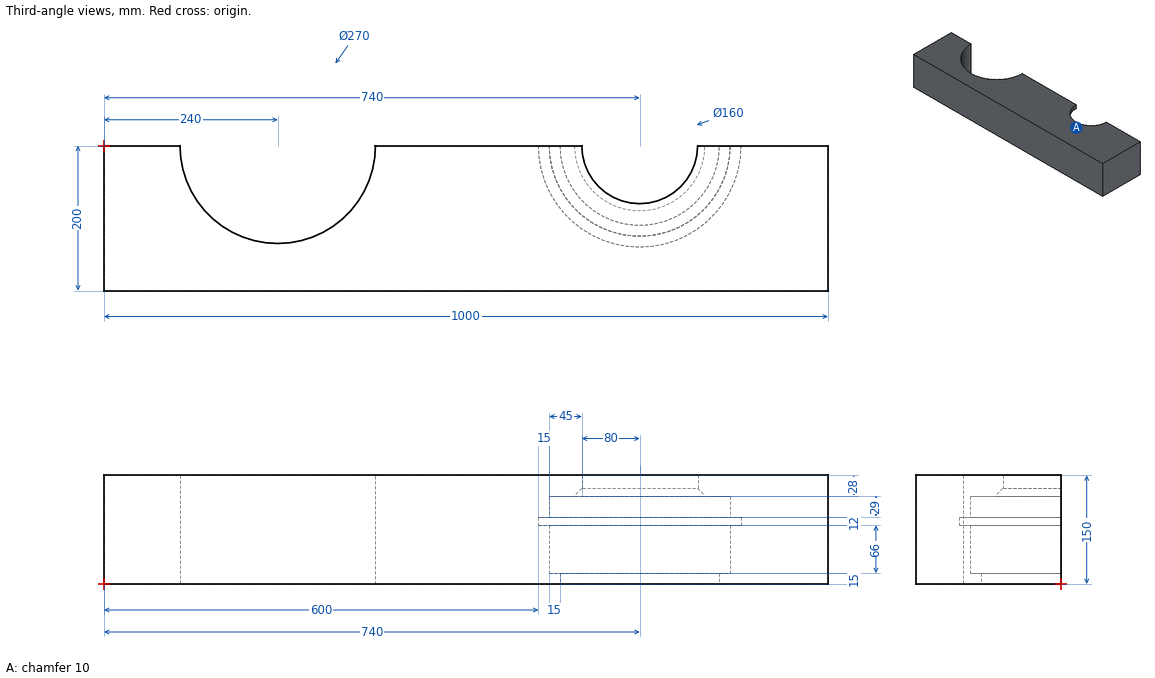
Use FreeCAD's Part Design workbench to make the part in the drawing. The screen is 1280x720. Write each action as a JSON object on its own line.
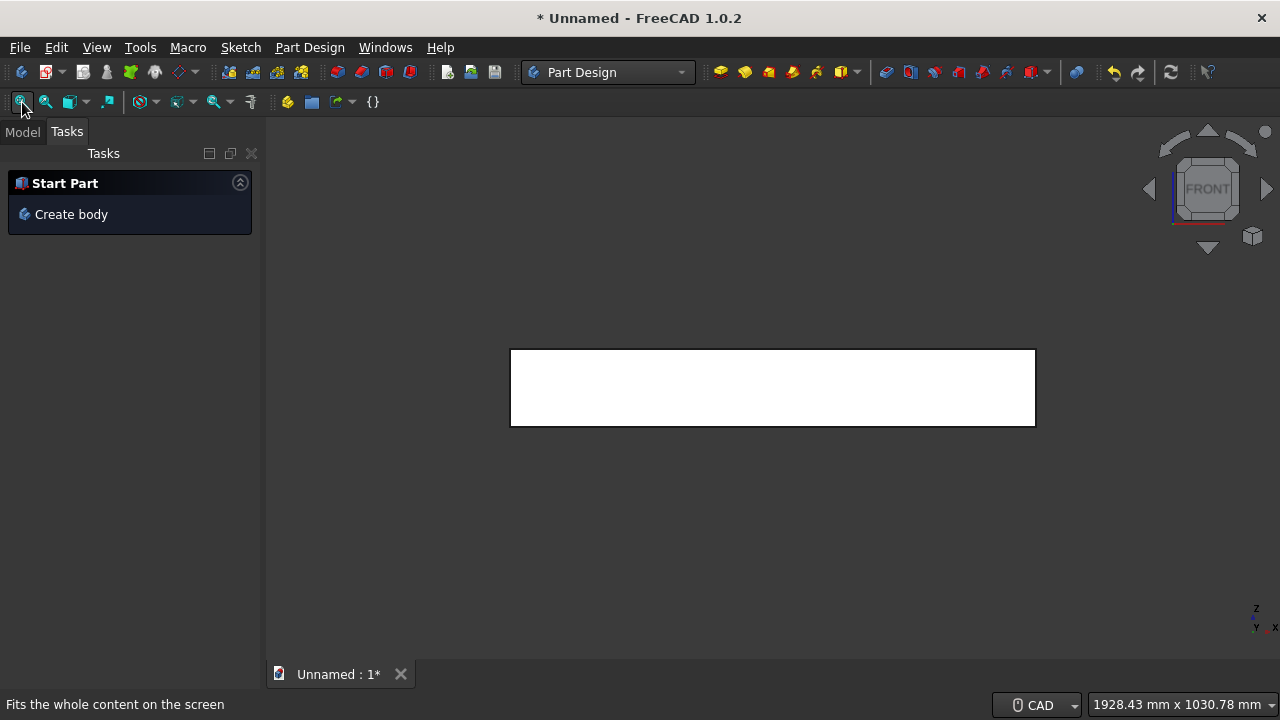
{"action": "key", "text": "3"}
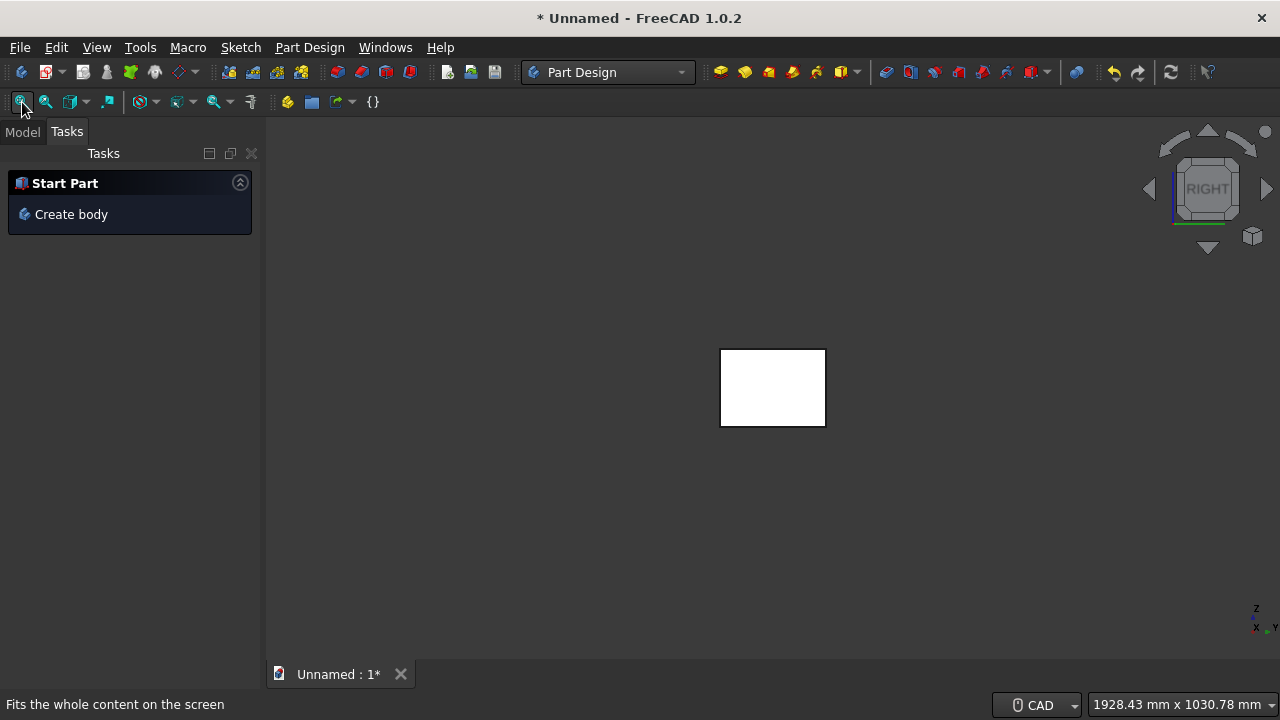
{"action": "left_click", "coordinate": [22, 102]}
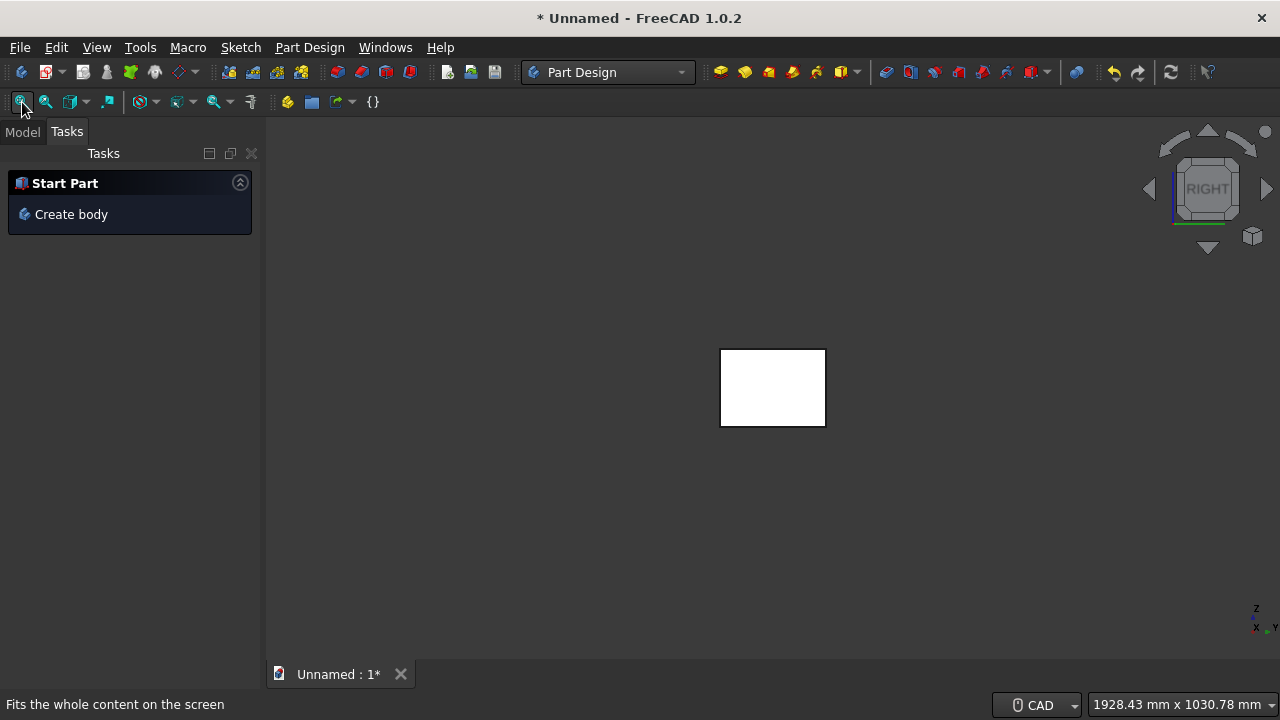
{"action": "key", "text": "5"}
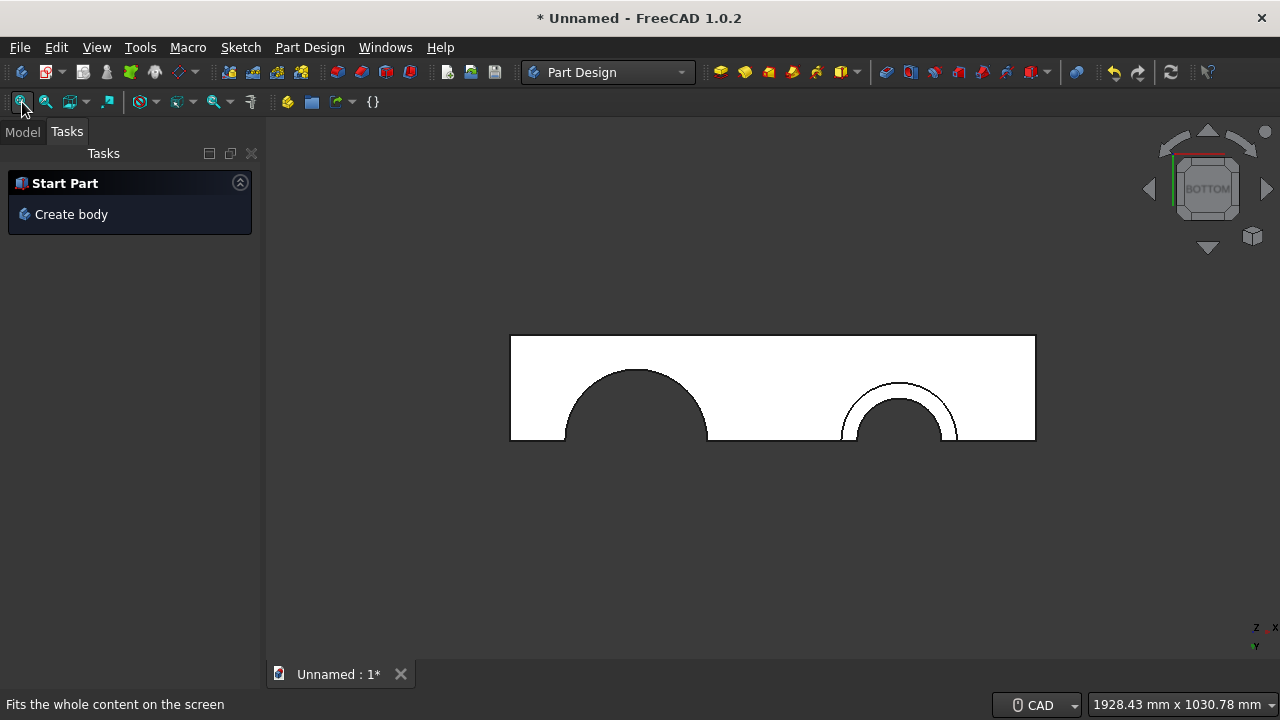
{"action": "left_click", "coordinate": [899, 398]}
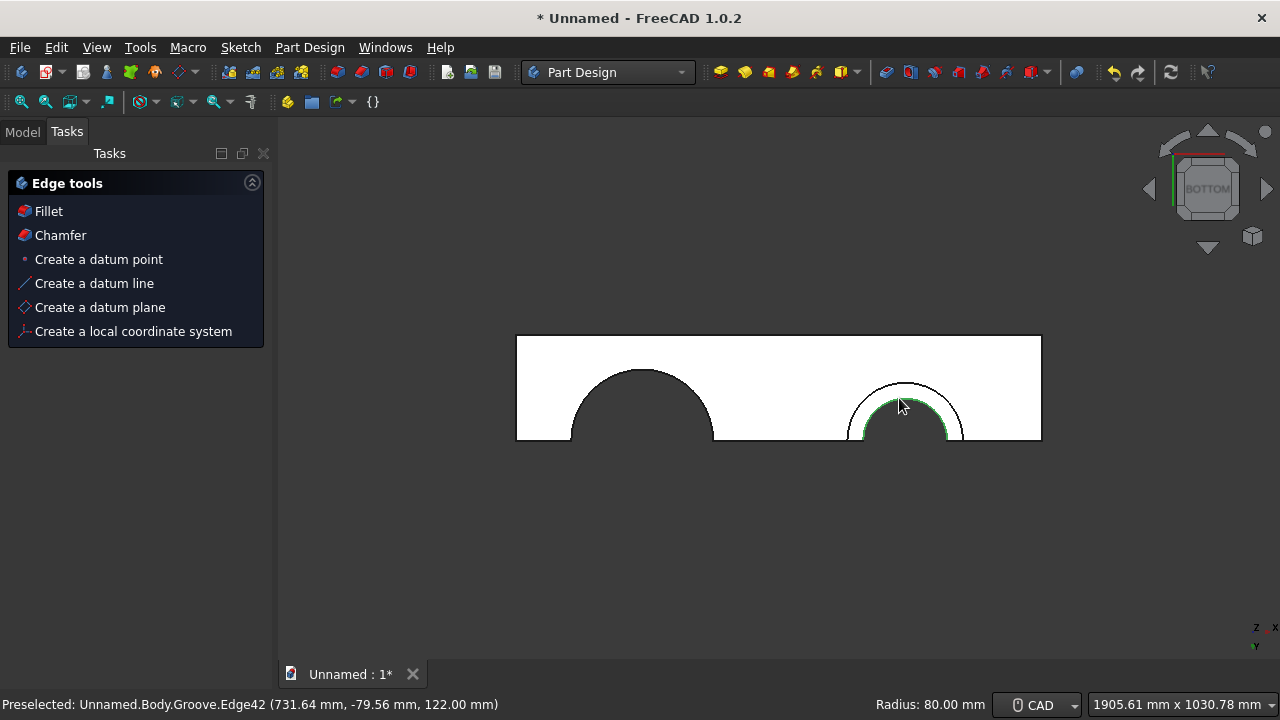
{"action": "left_click", "coordinate": [362, 72]}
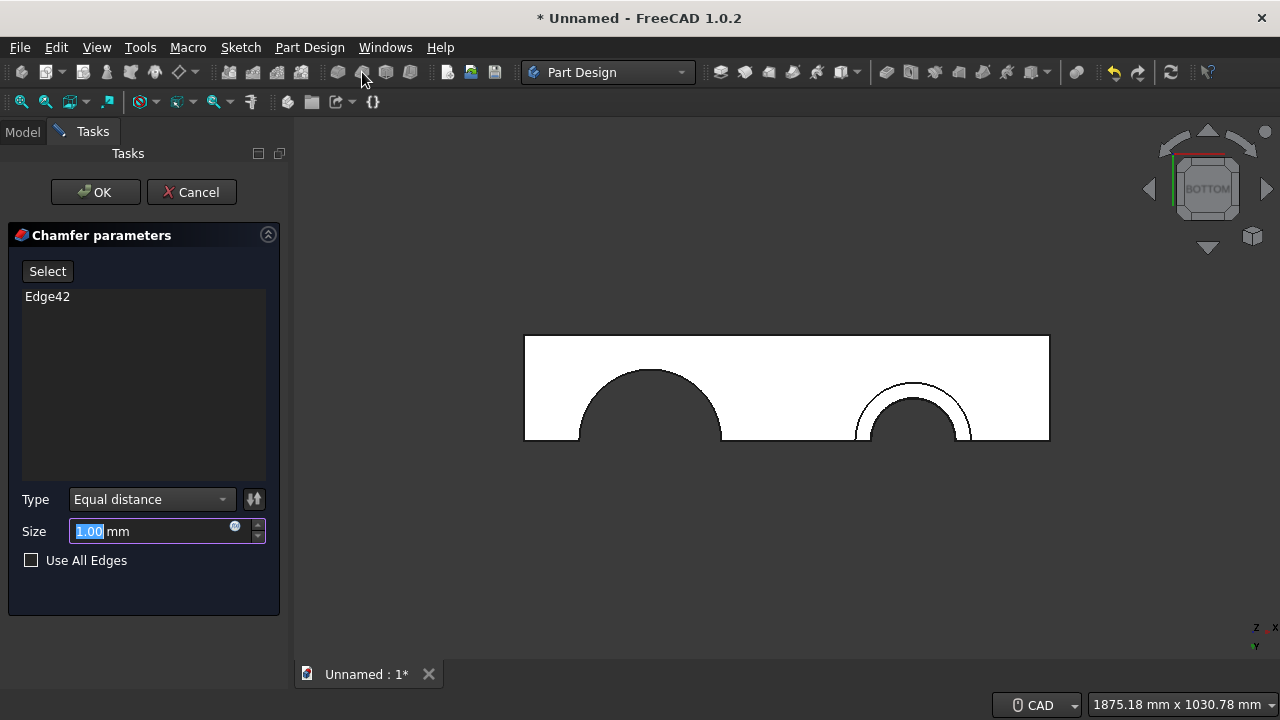
{"action": "type", "text": "10"}
{"action": "key", "text": "Tab"}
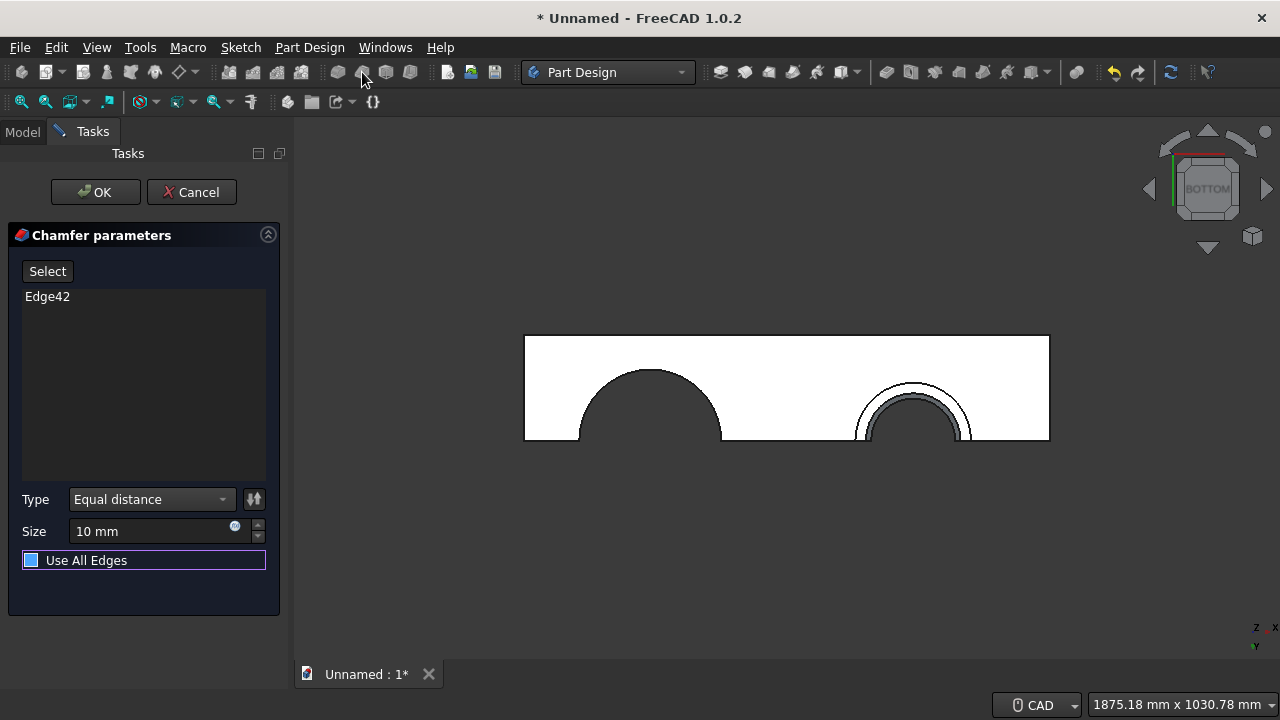
{"action": "left_click", "coordinate": [96, 192]}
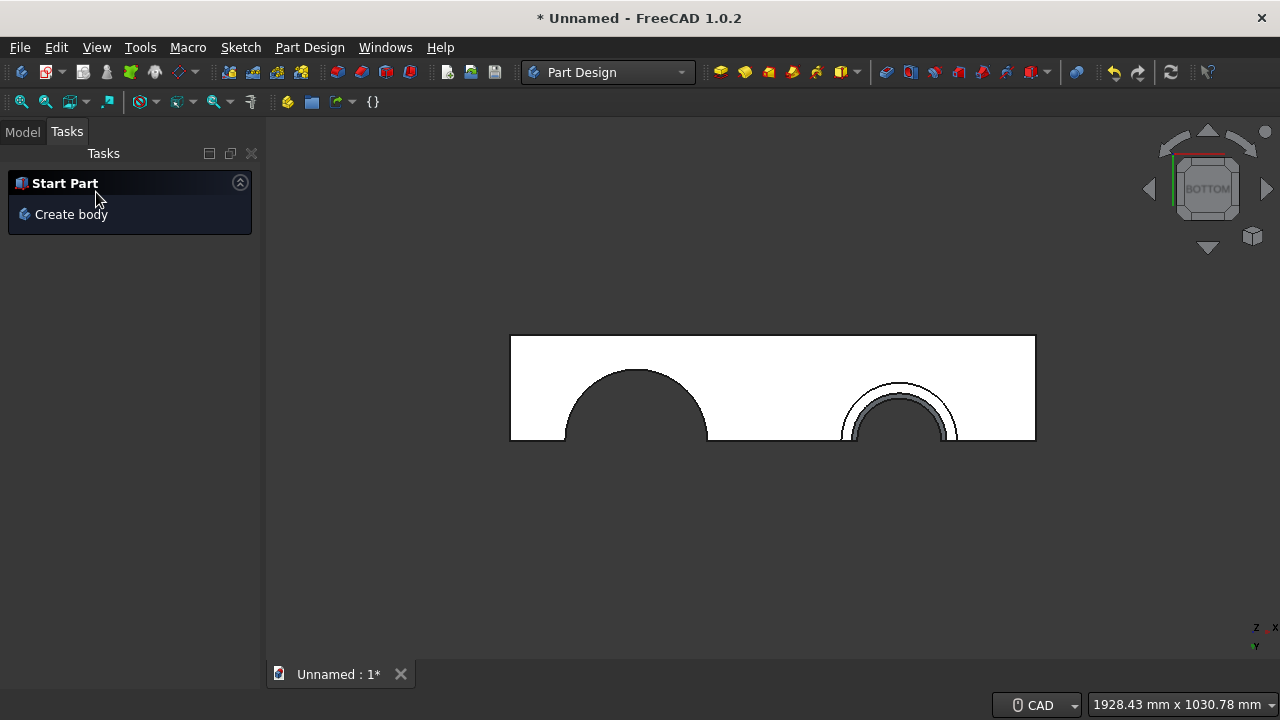
{"action": "key", "text": "0"}